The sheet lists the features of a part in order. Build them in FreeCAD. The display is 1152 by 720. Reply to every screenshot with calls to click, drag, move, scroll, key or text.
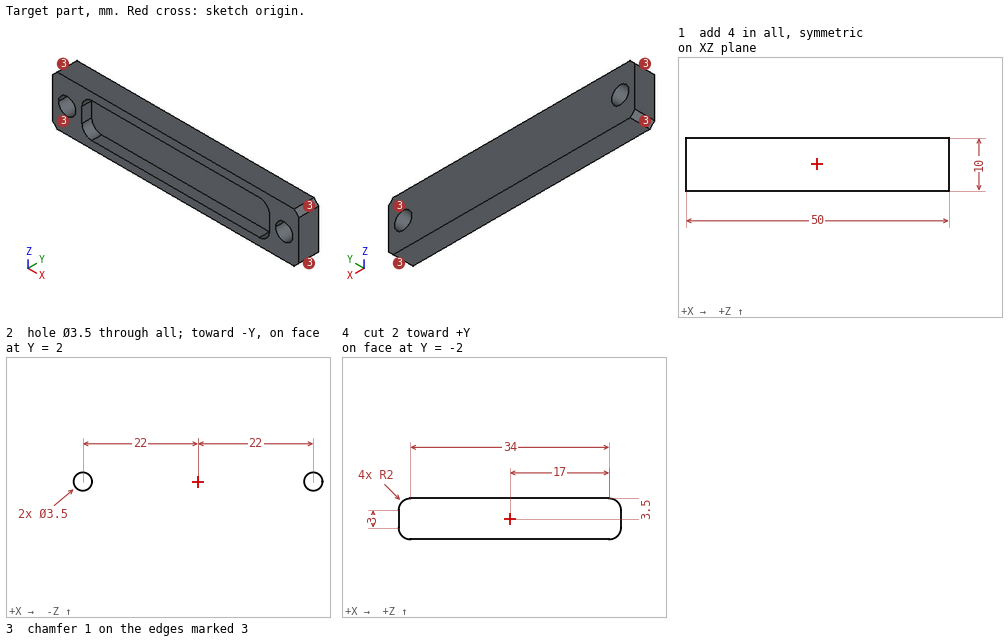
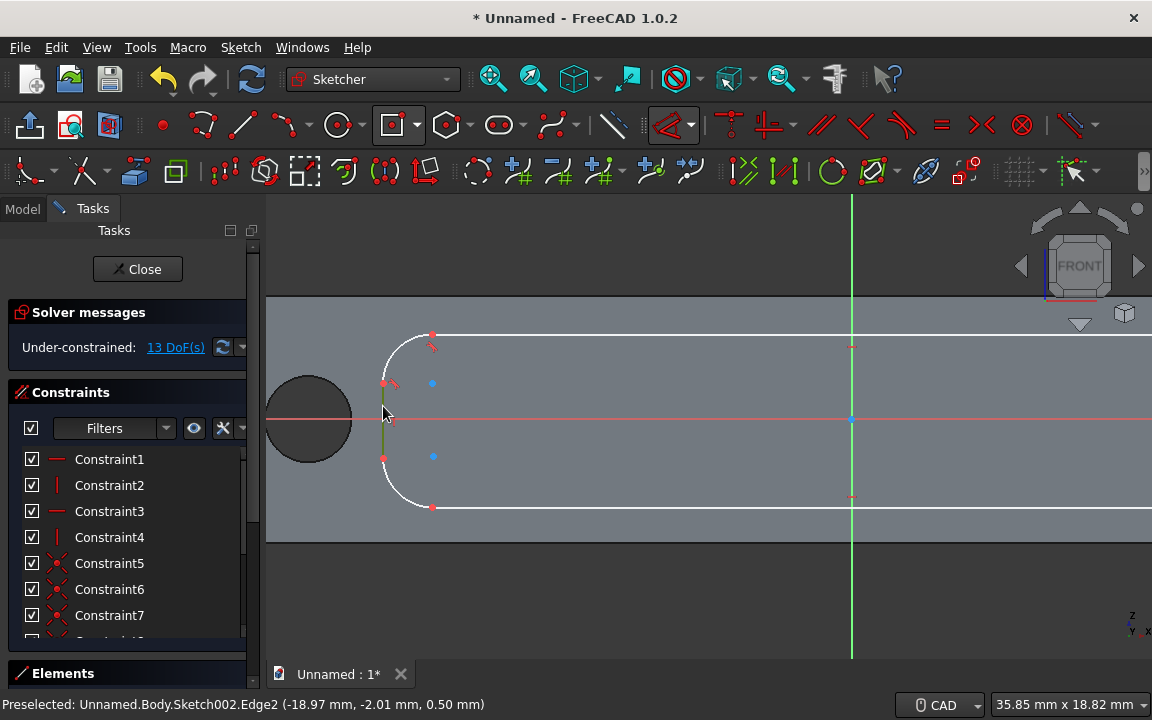
click(389, 480)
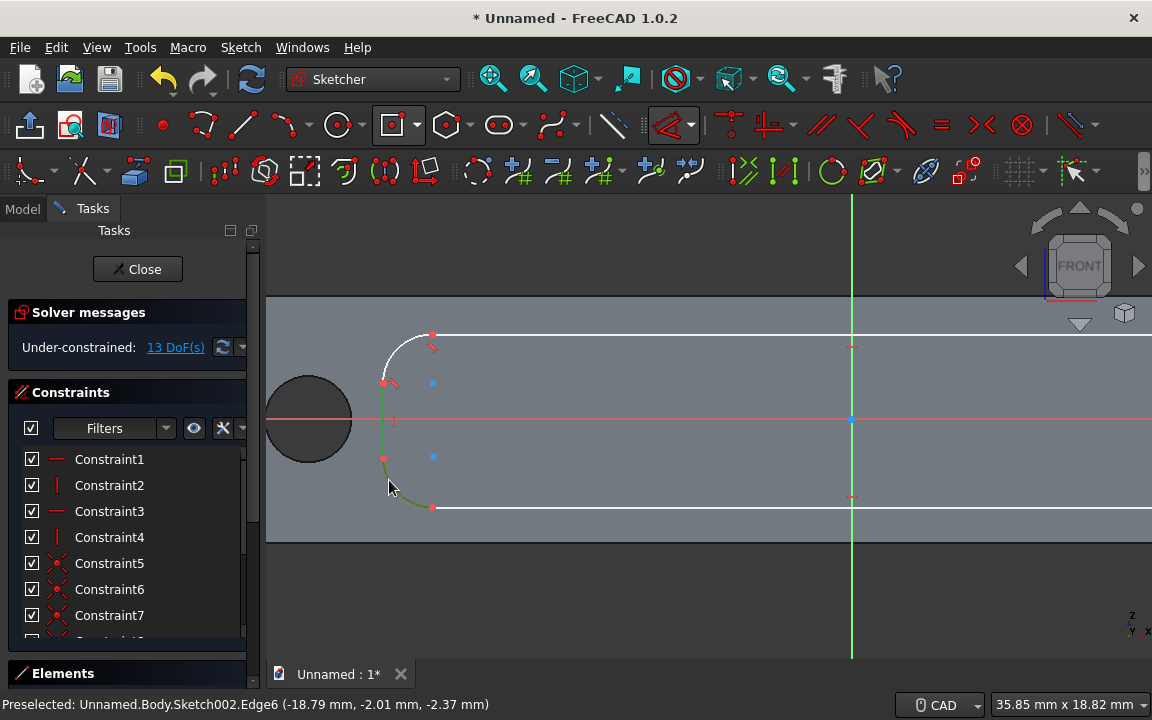
click(902, 126)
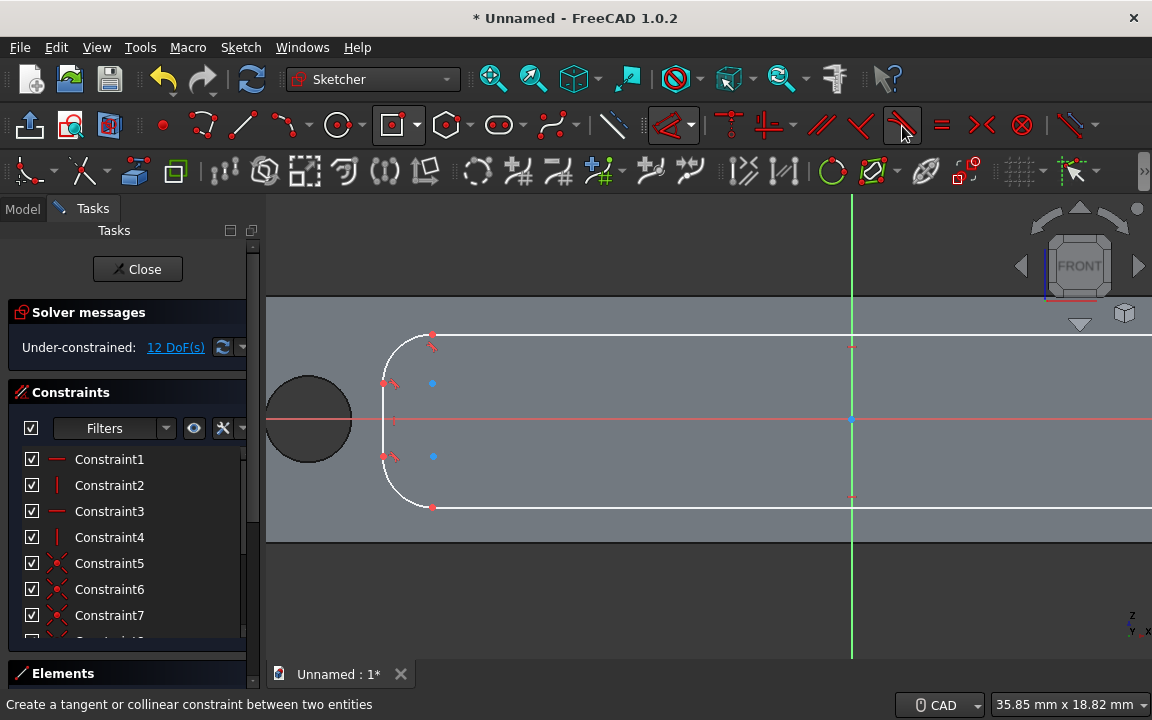
click(684, 508)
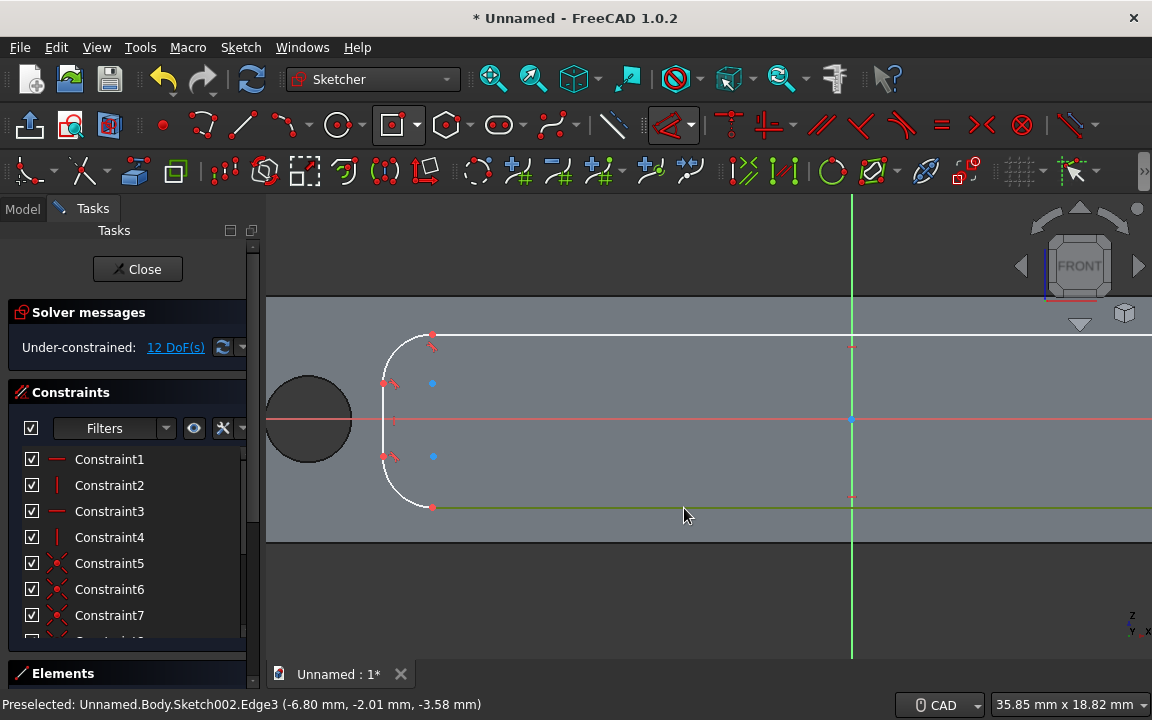
click(388, 480)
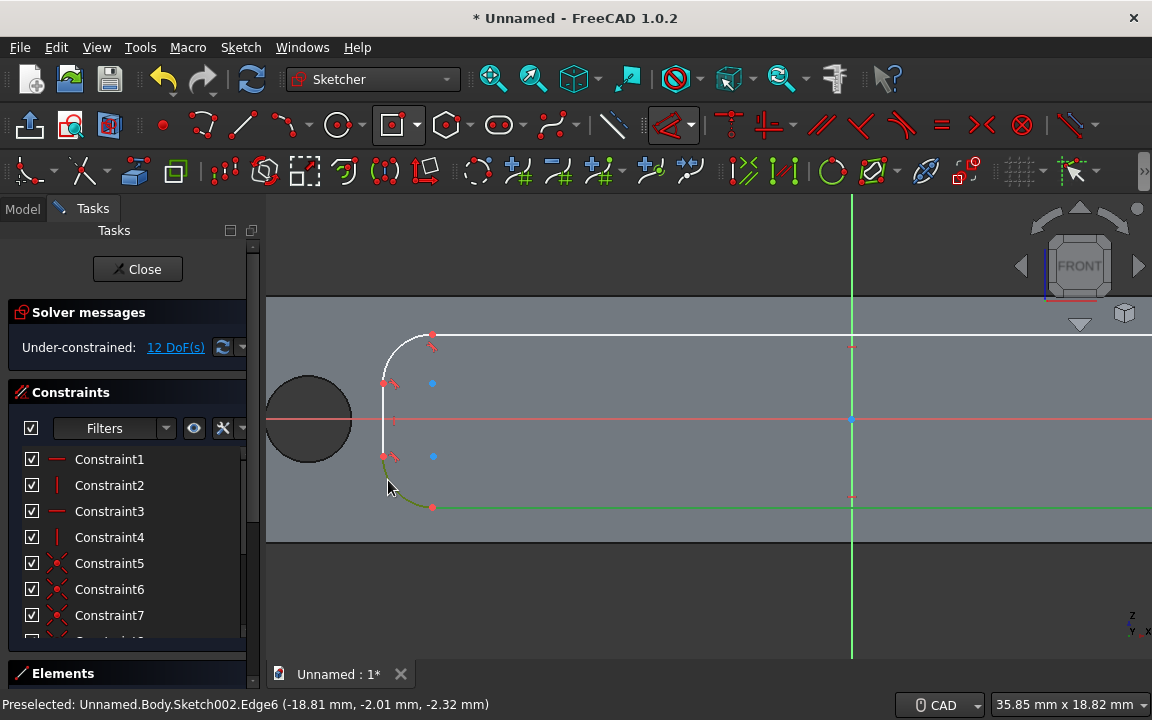
click(902, 126)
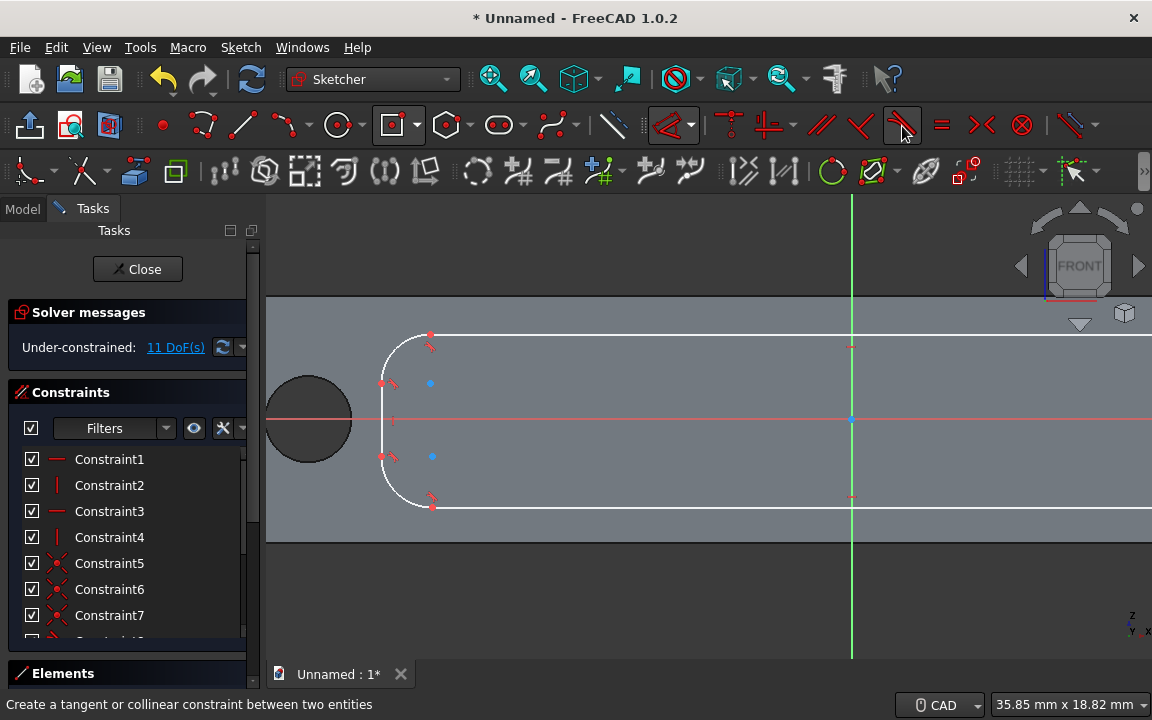
click(684, 508)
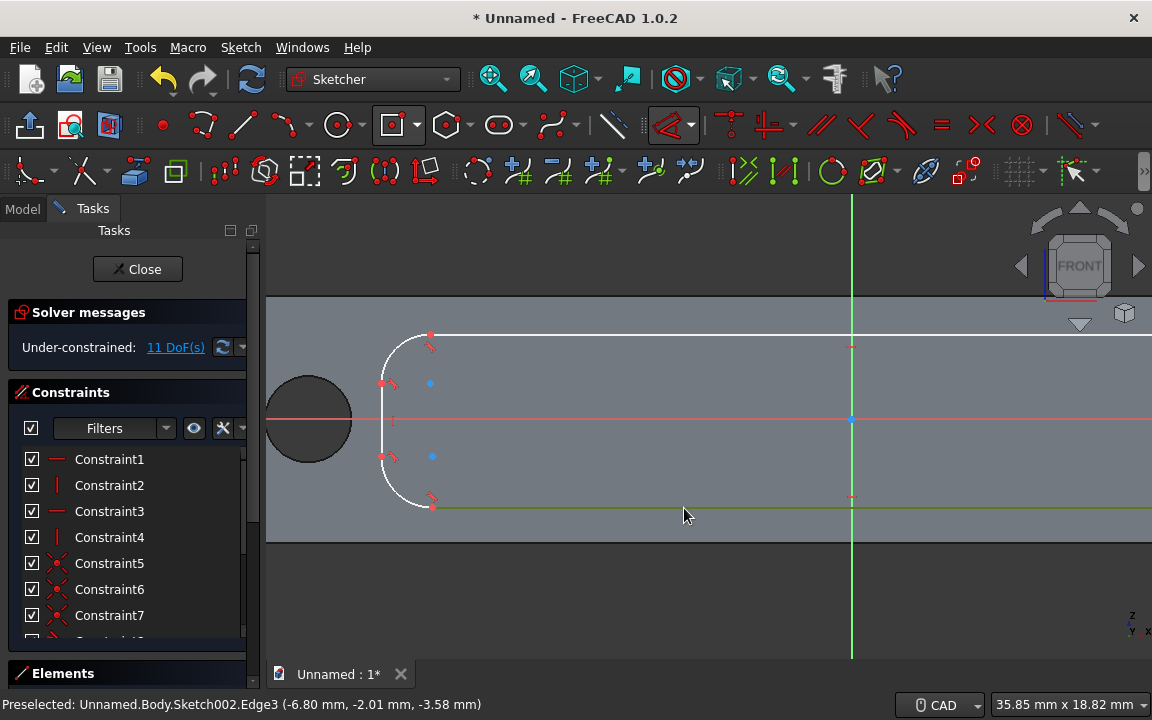
scroll(383, 435, down, 3)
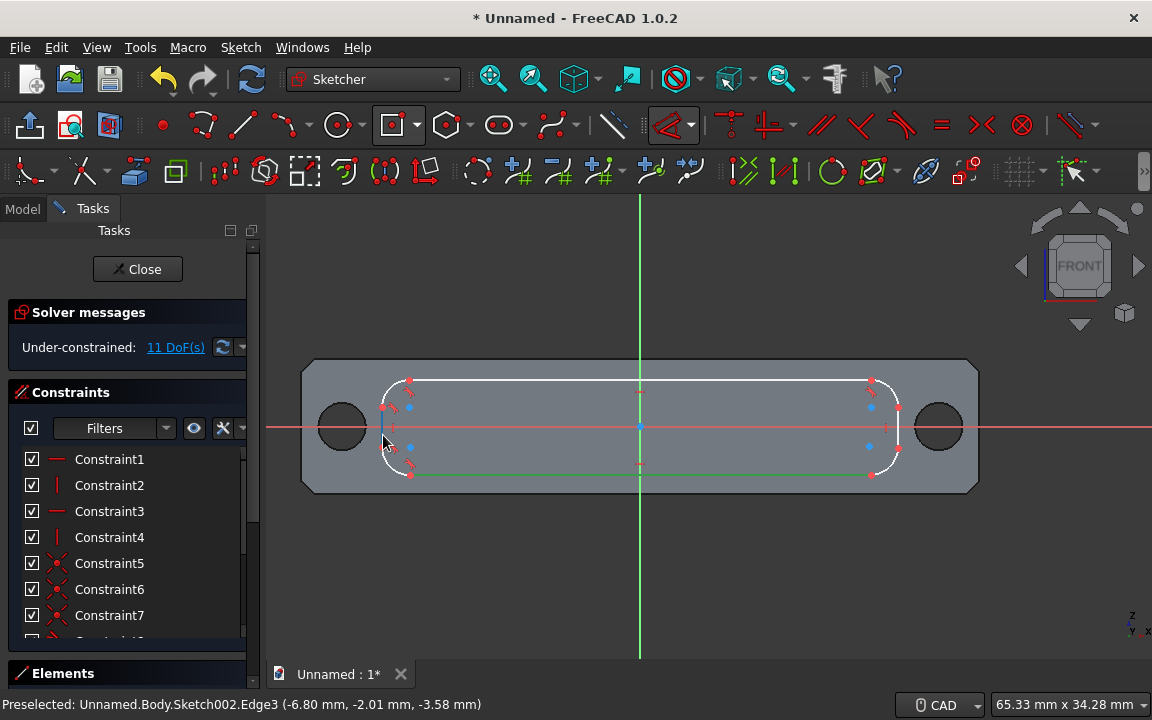
click(883, 472)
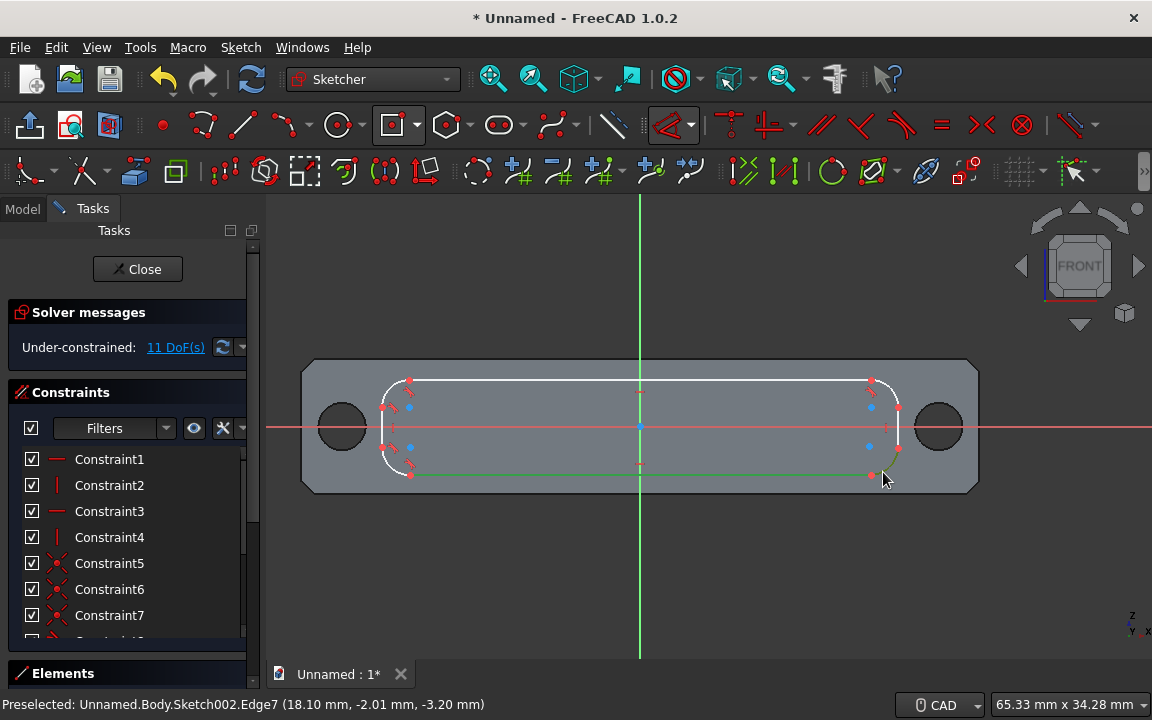
click(902, 126)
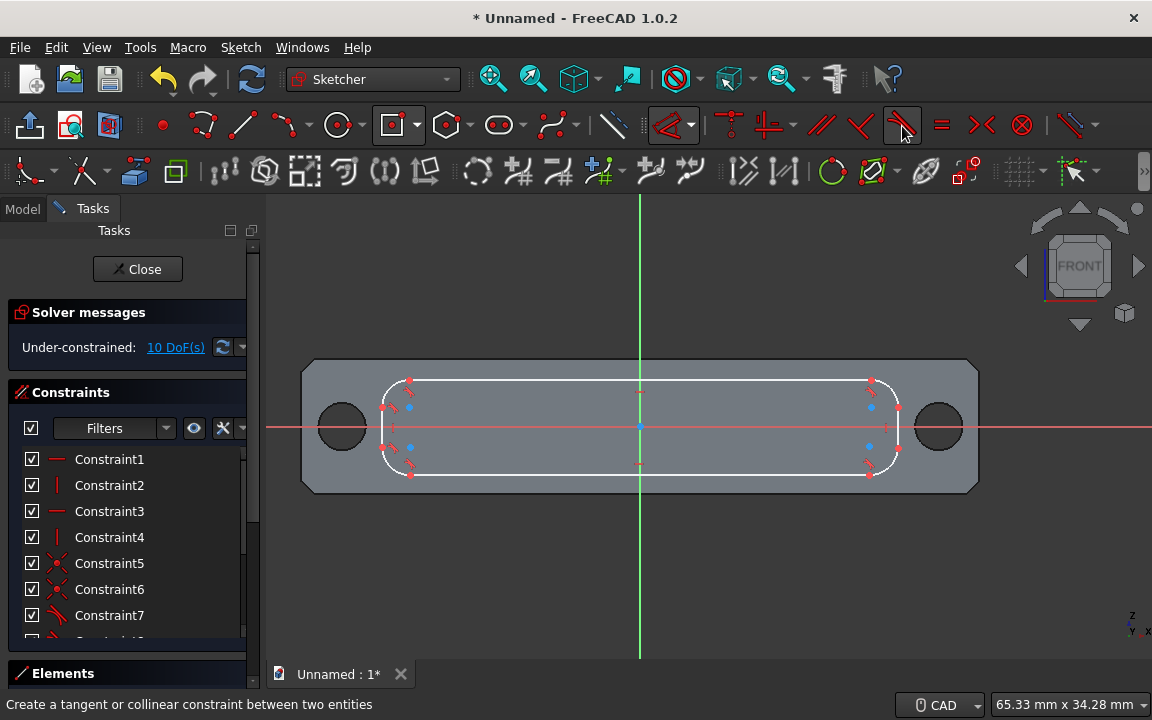
scroll(898, 436, up, 3)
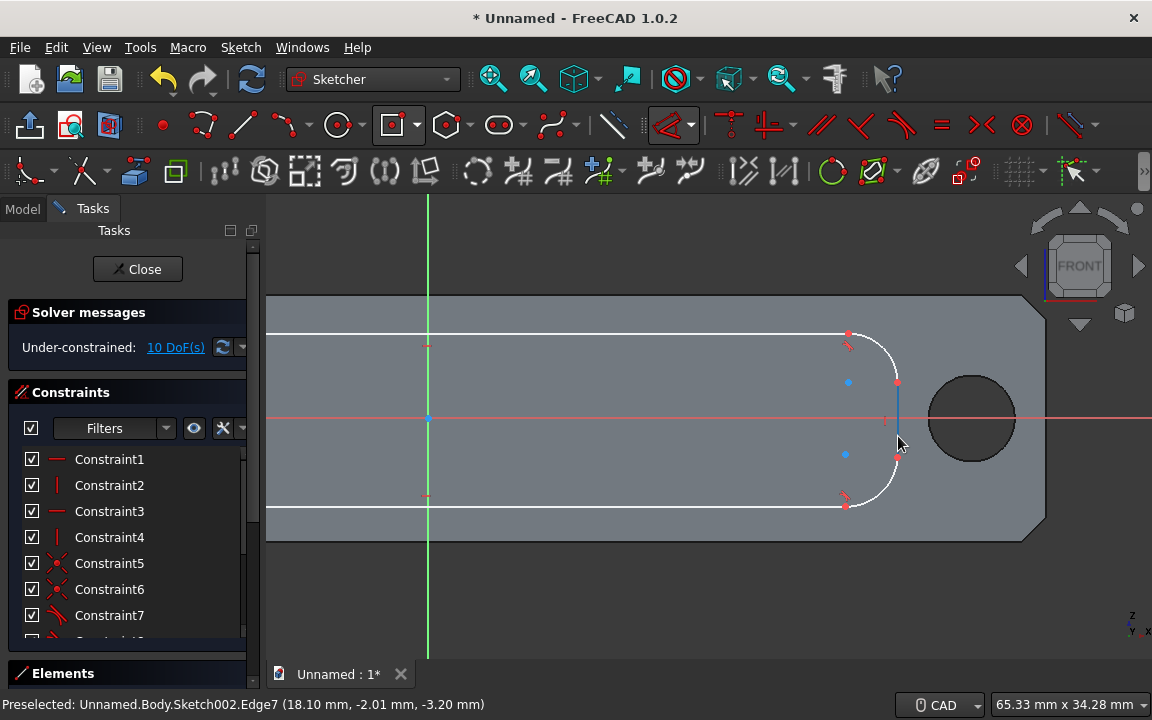
click(898, 435)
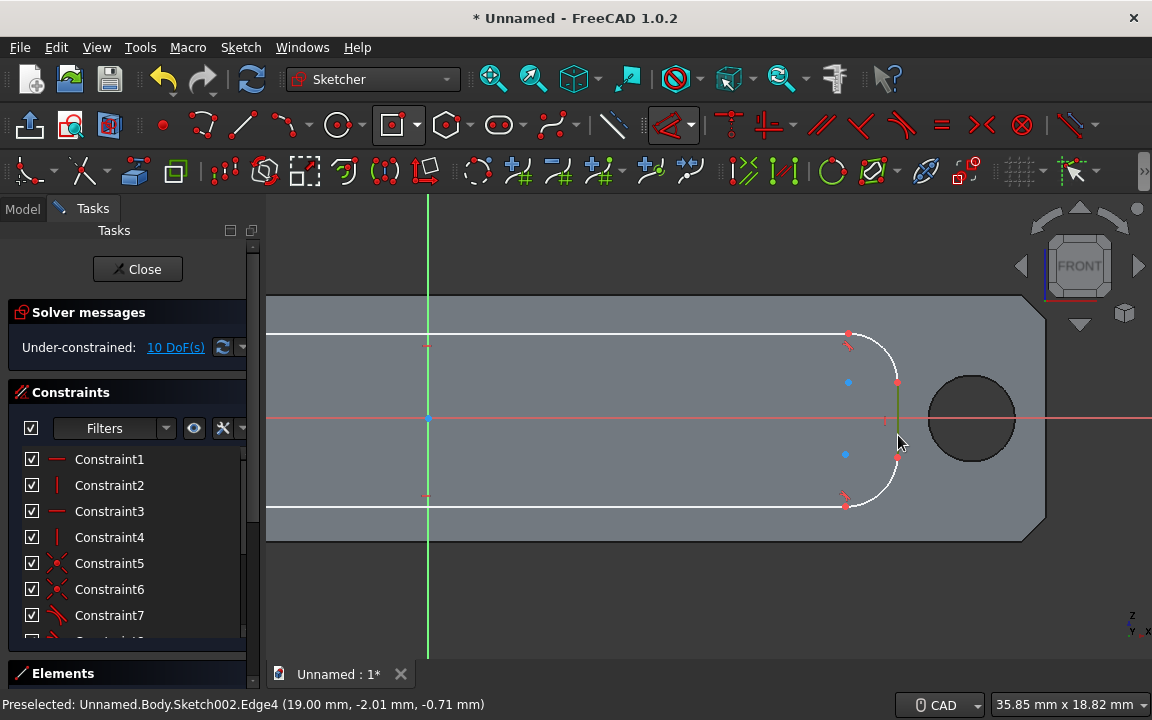
click(868, 502)